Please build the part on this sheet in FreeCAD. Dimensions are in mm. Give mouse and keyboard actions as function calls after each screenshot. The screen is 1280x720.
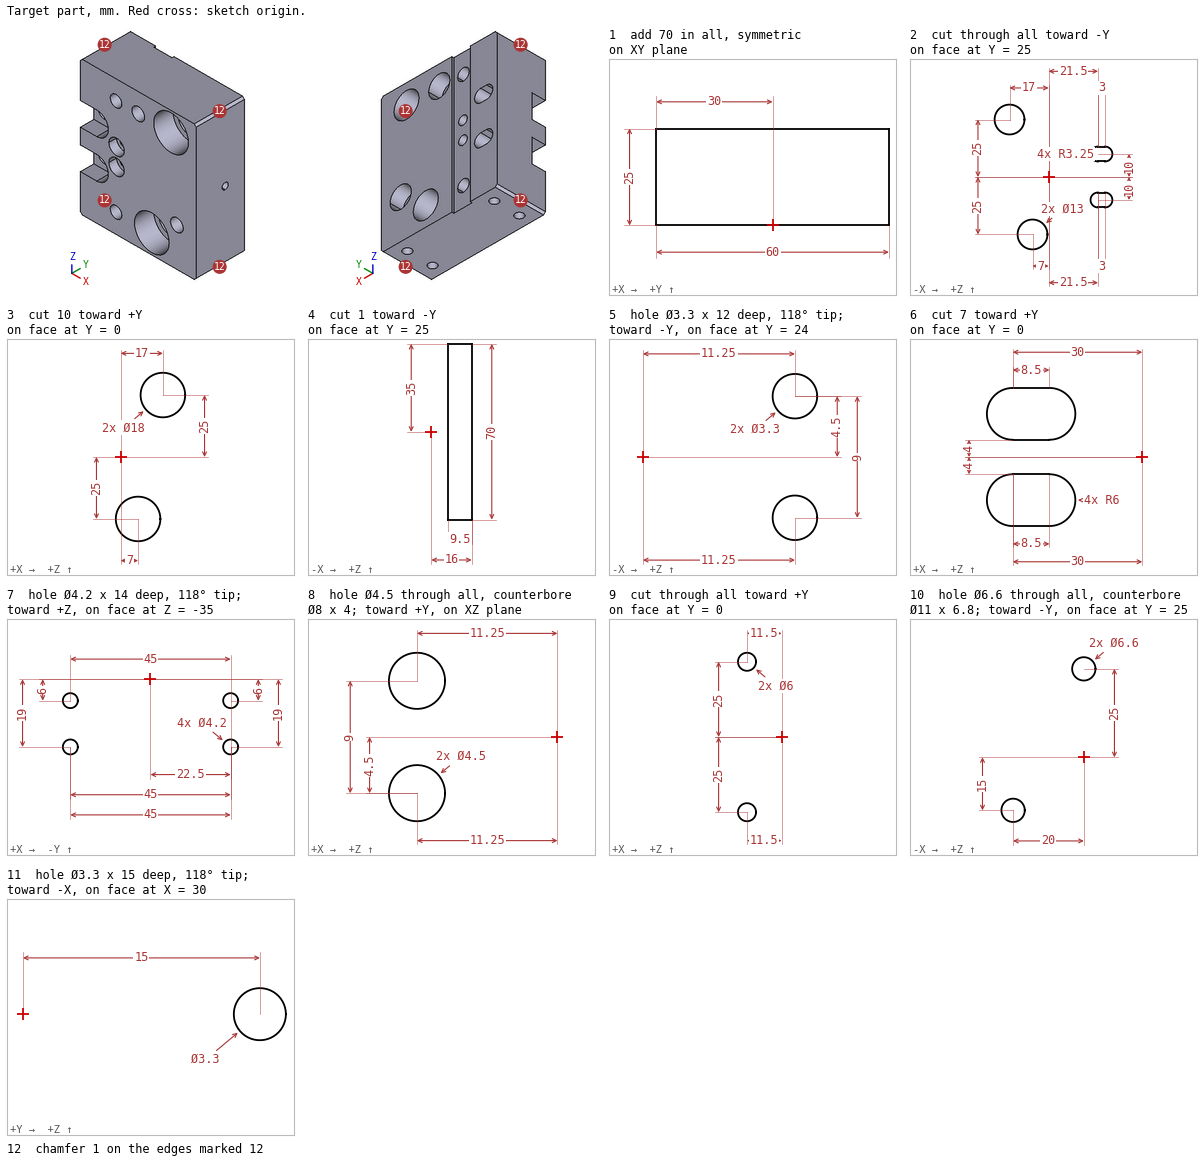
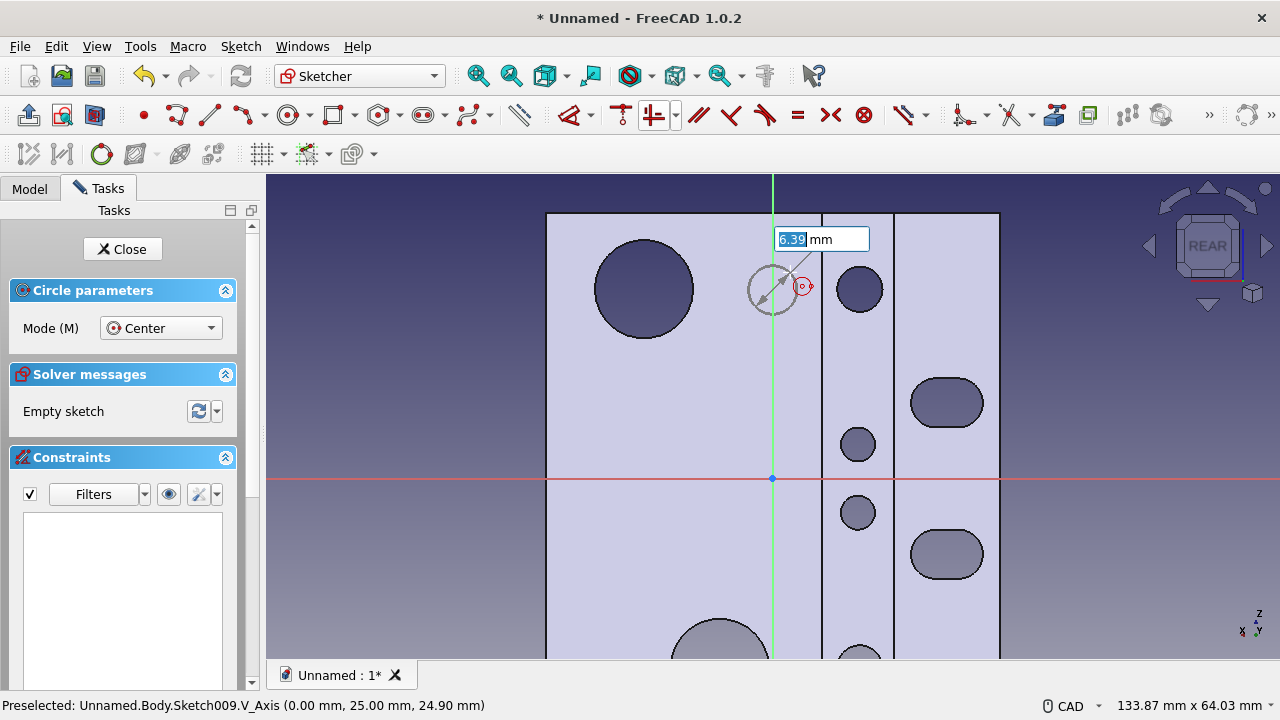
text(6.6)
key(Return)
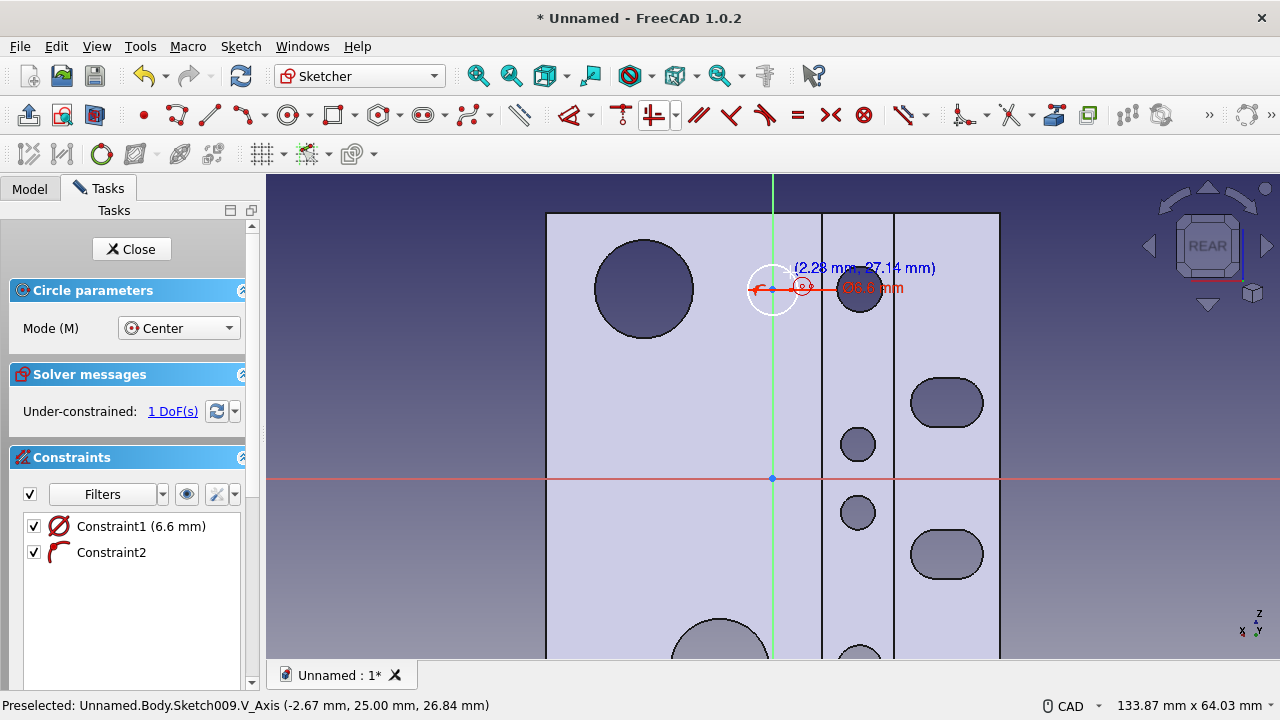
click(621, 592)
move(639, 575)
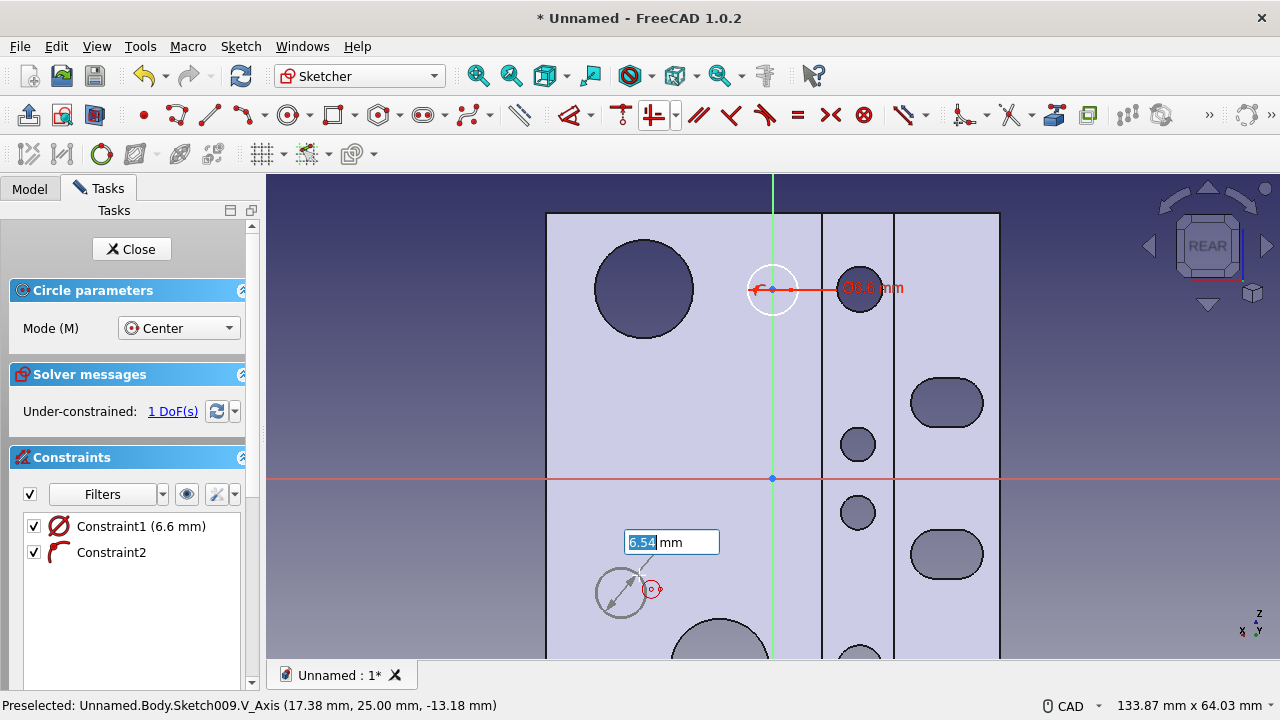
text(6.6)
key(Return)
key(Escape)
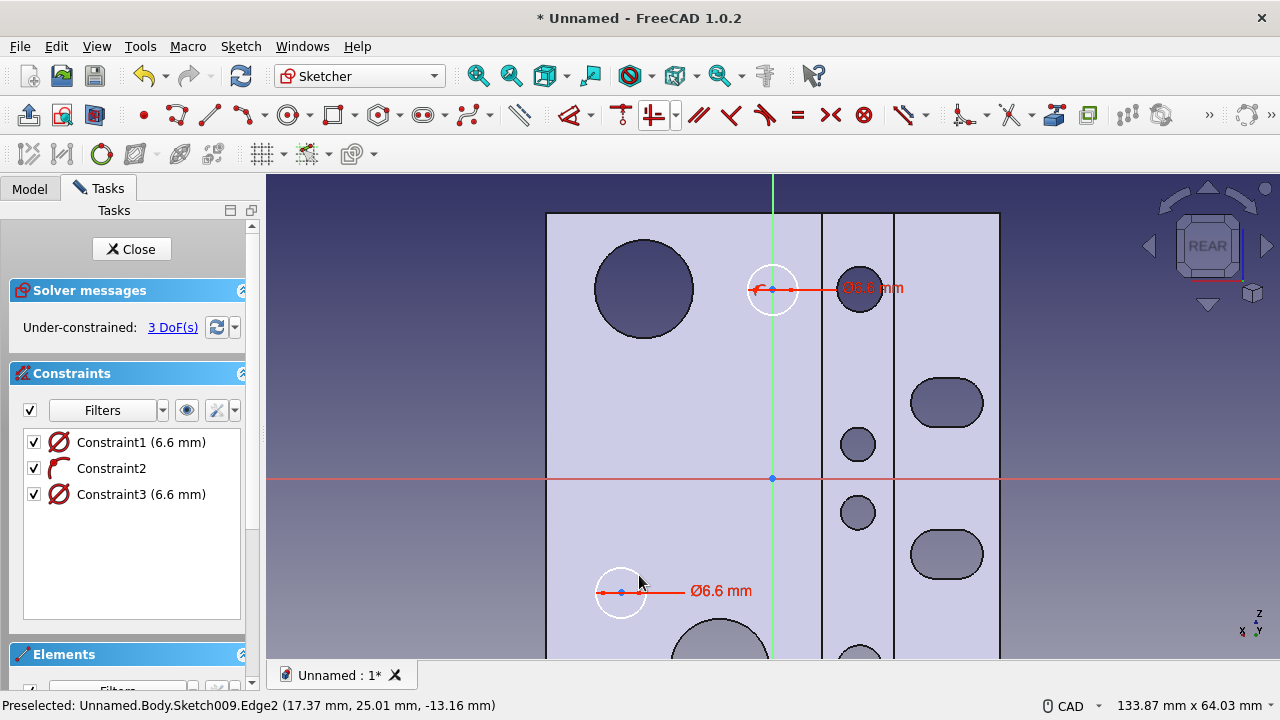
click(568, 116)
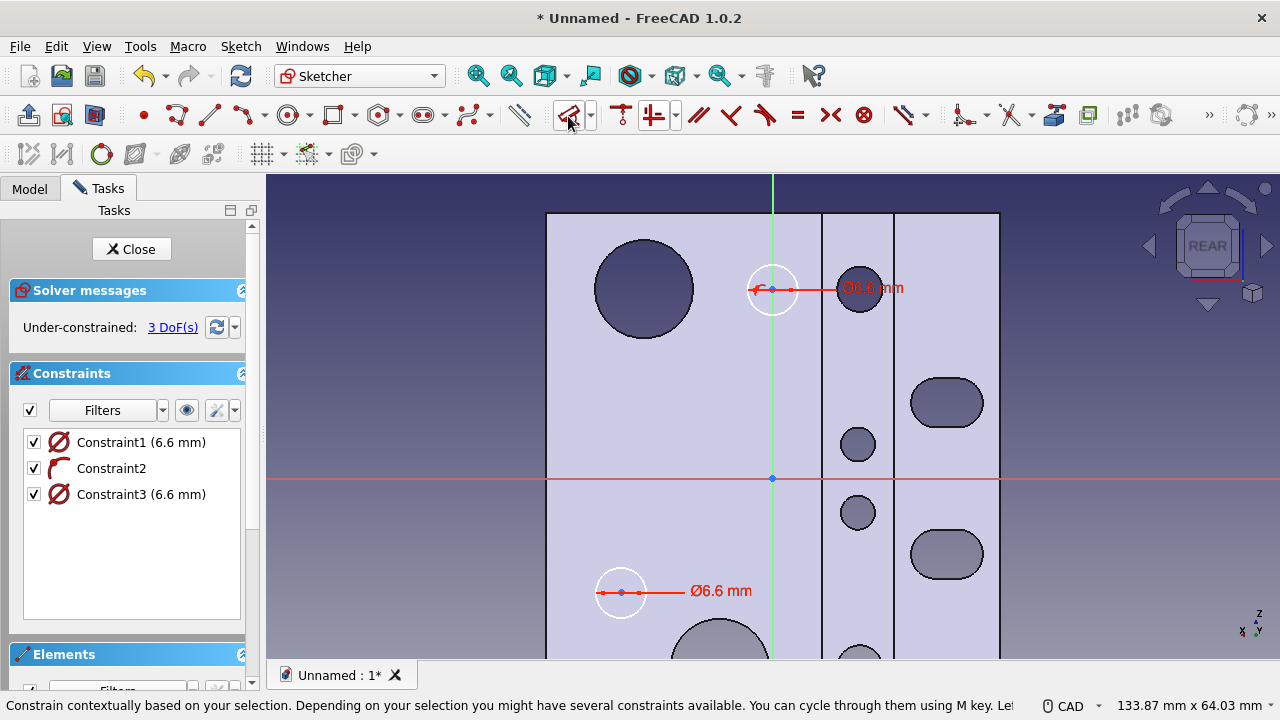
click(773, 290)
click(807, 384)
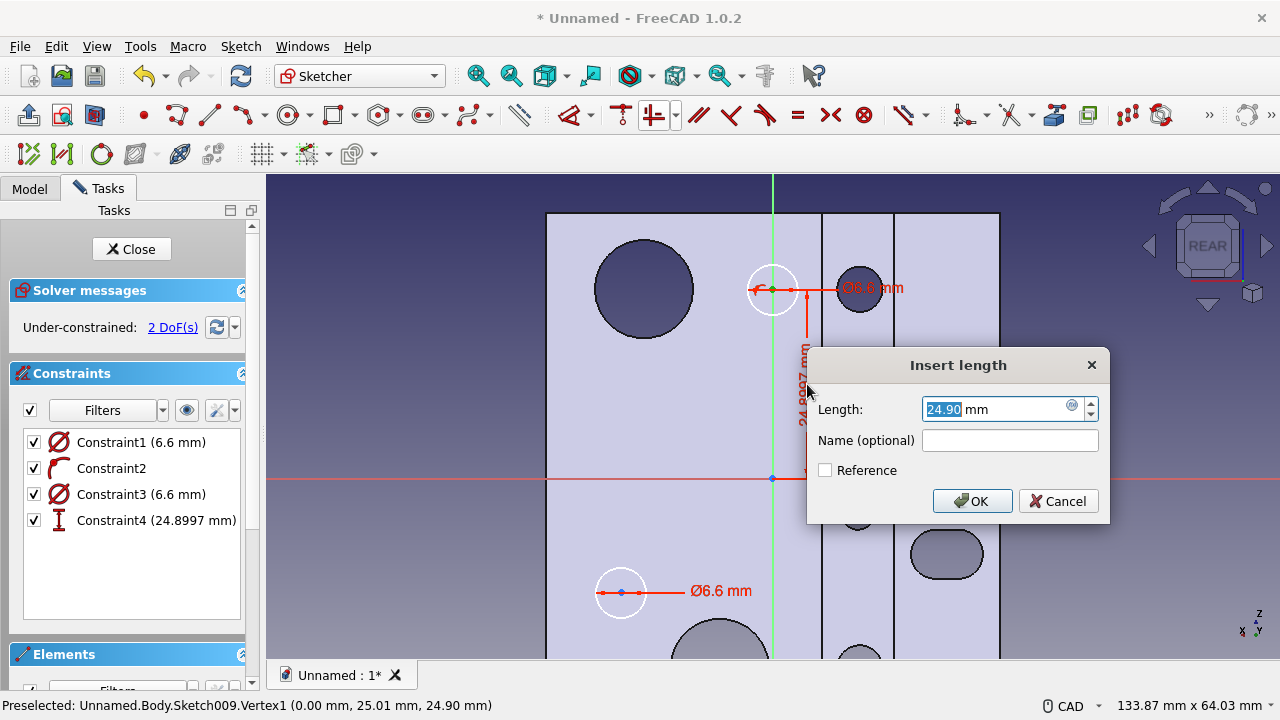
text(25)
key(Return)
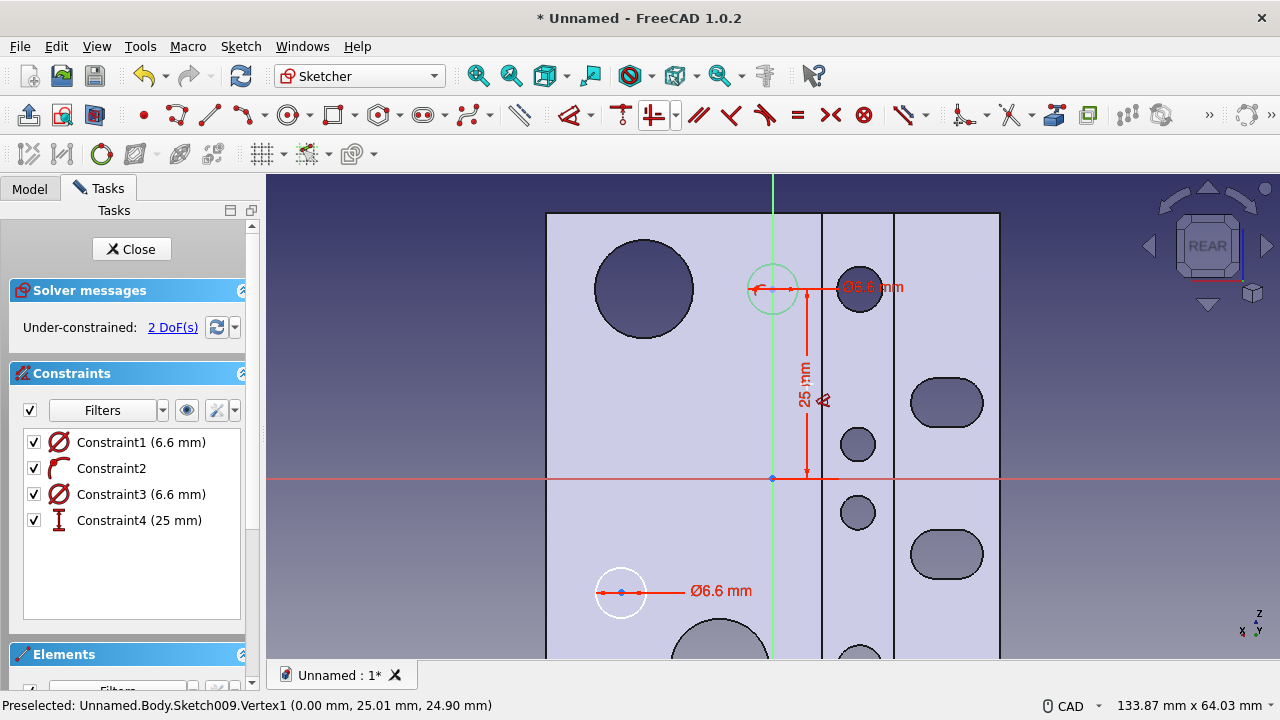
click(621, 593)
click(697, 627)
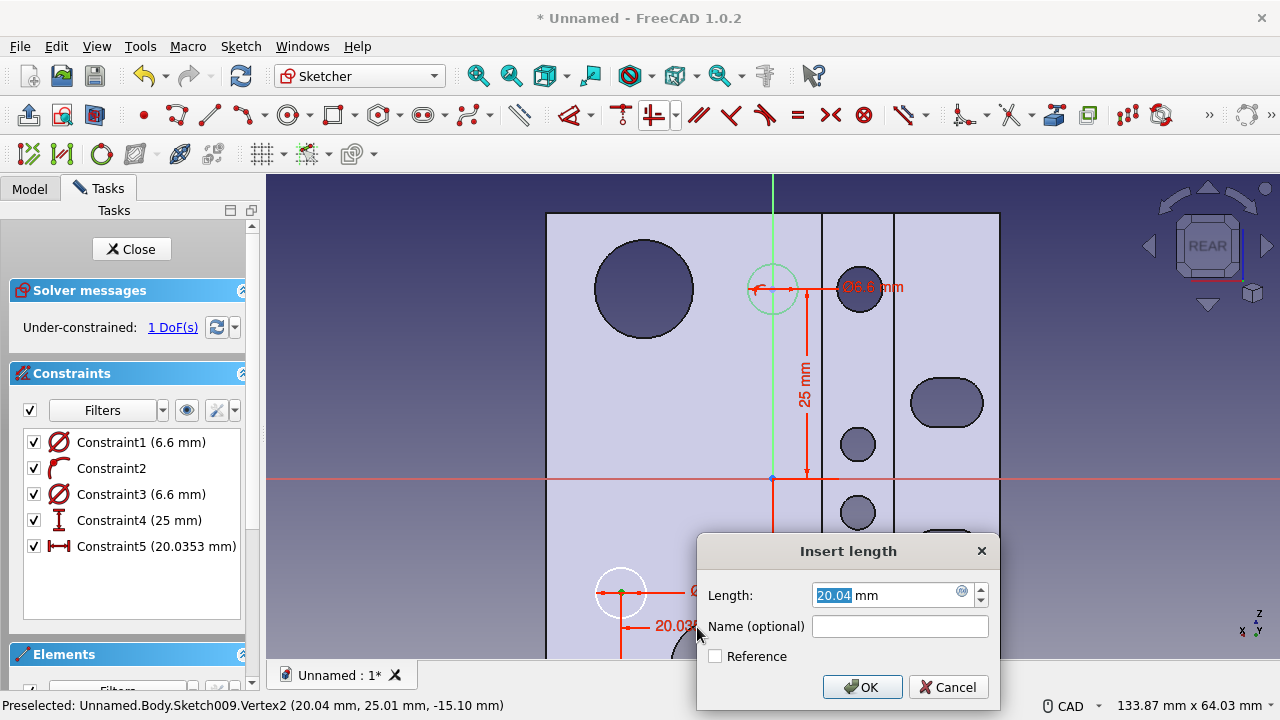
text(20)
key(Return)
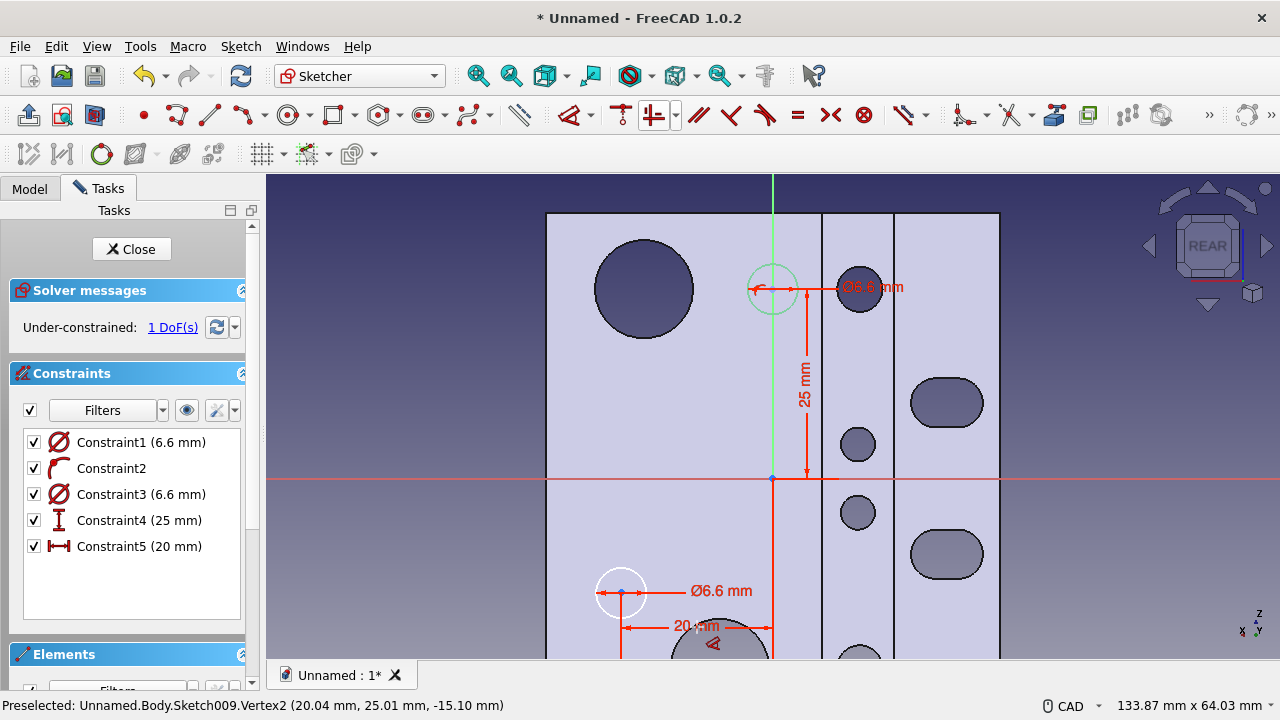
click(621, 593)
click(807, 536)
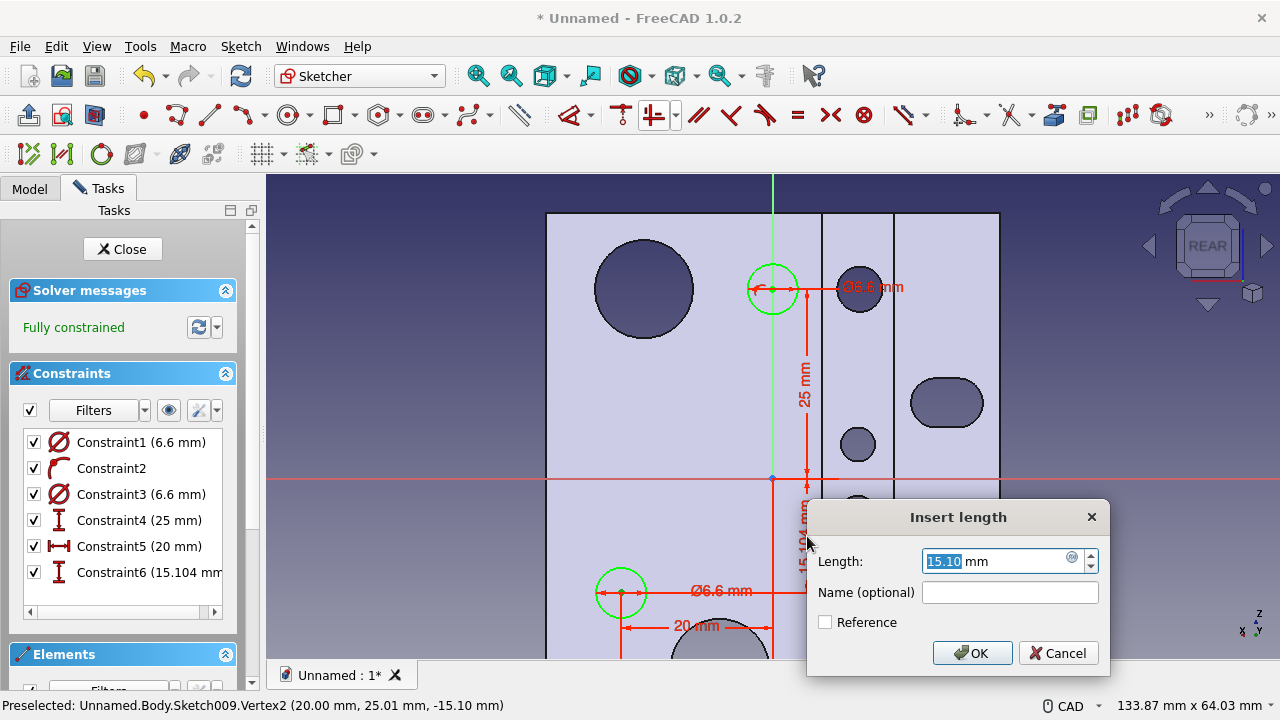
text(15)
key(Return)
key(Escape)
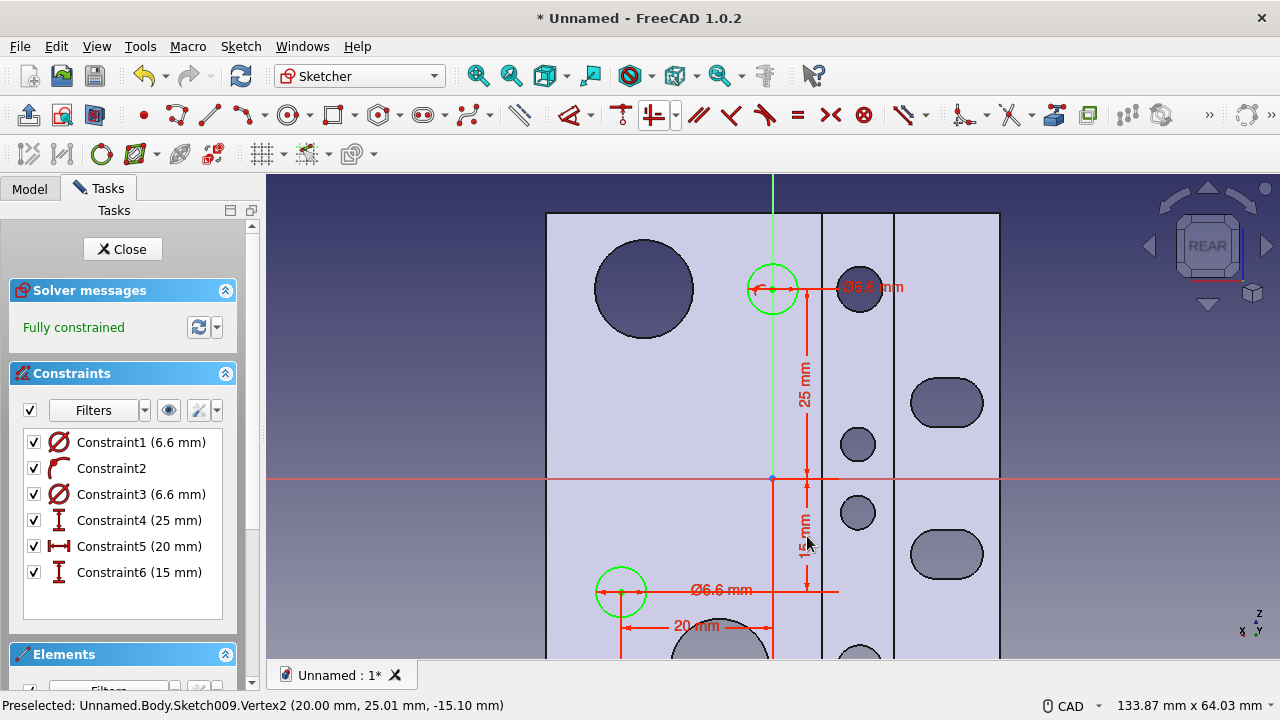
click(123, 249)